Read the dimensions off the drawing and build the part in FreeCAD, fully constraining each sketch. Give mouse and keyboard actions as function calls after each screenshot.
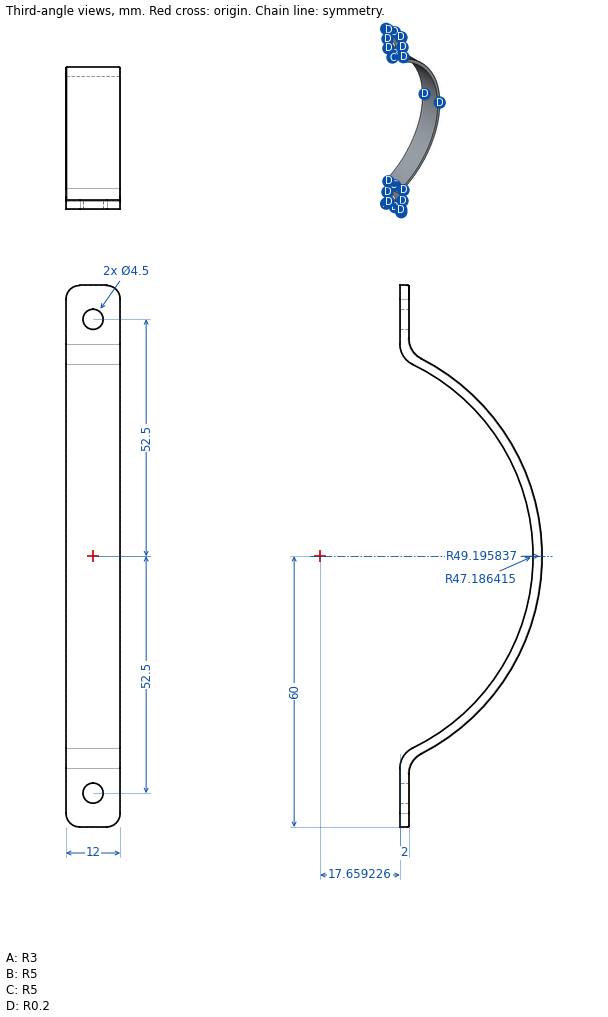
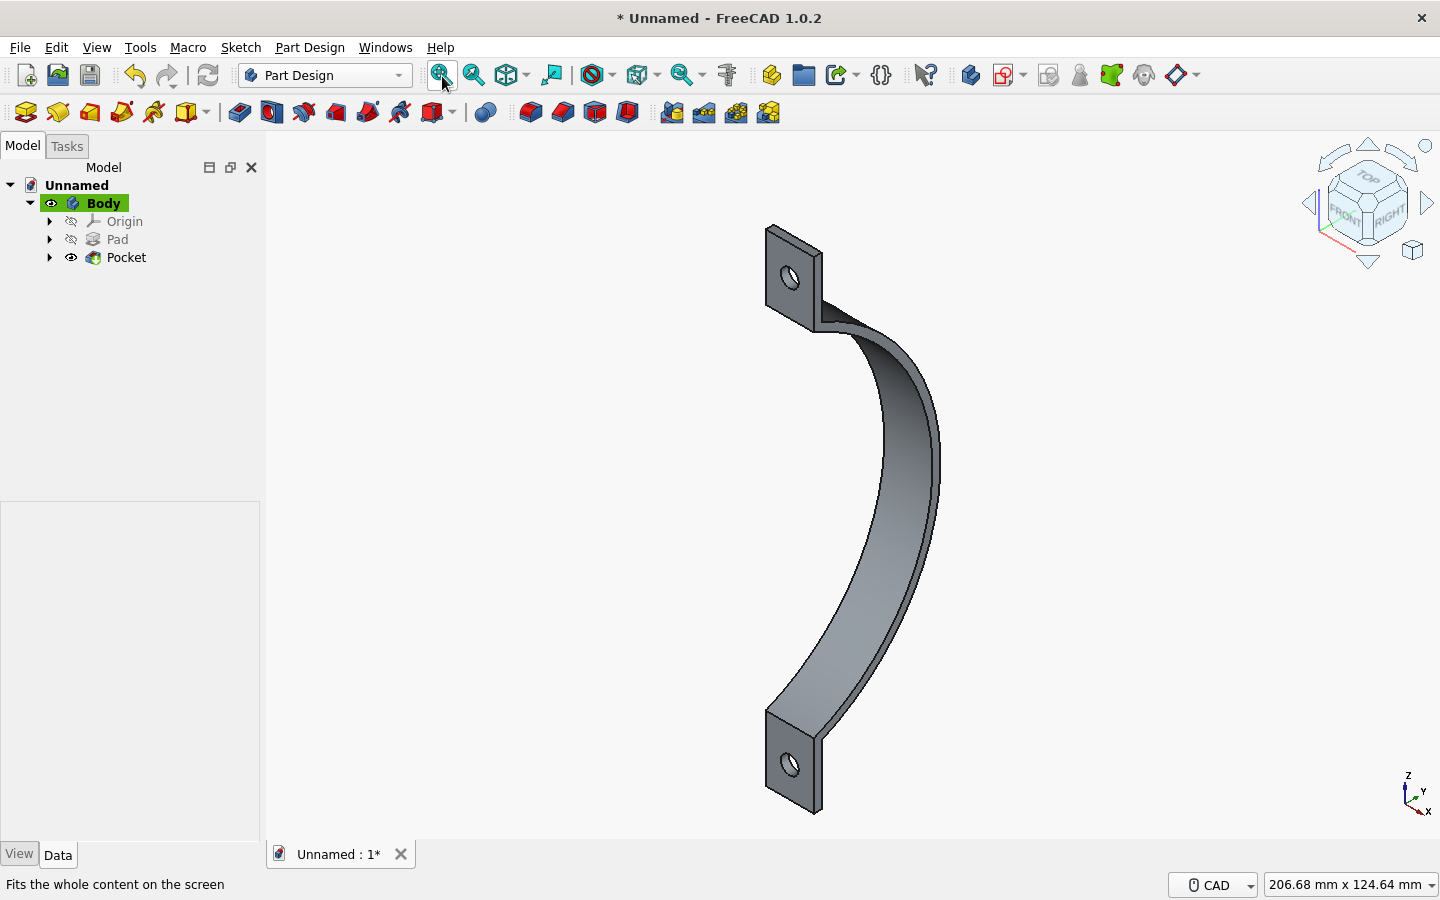
key(2)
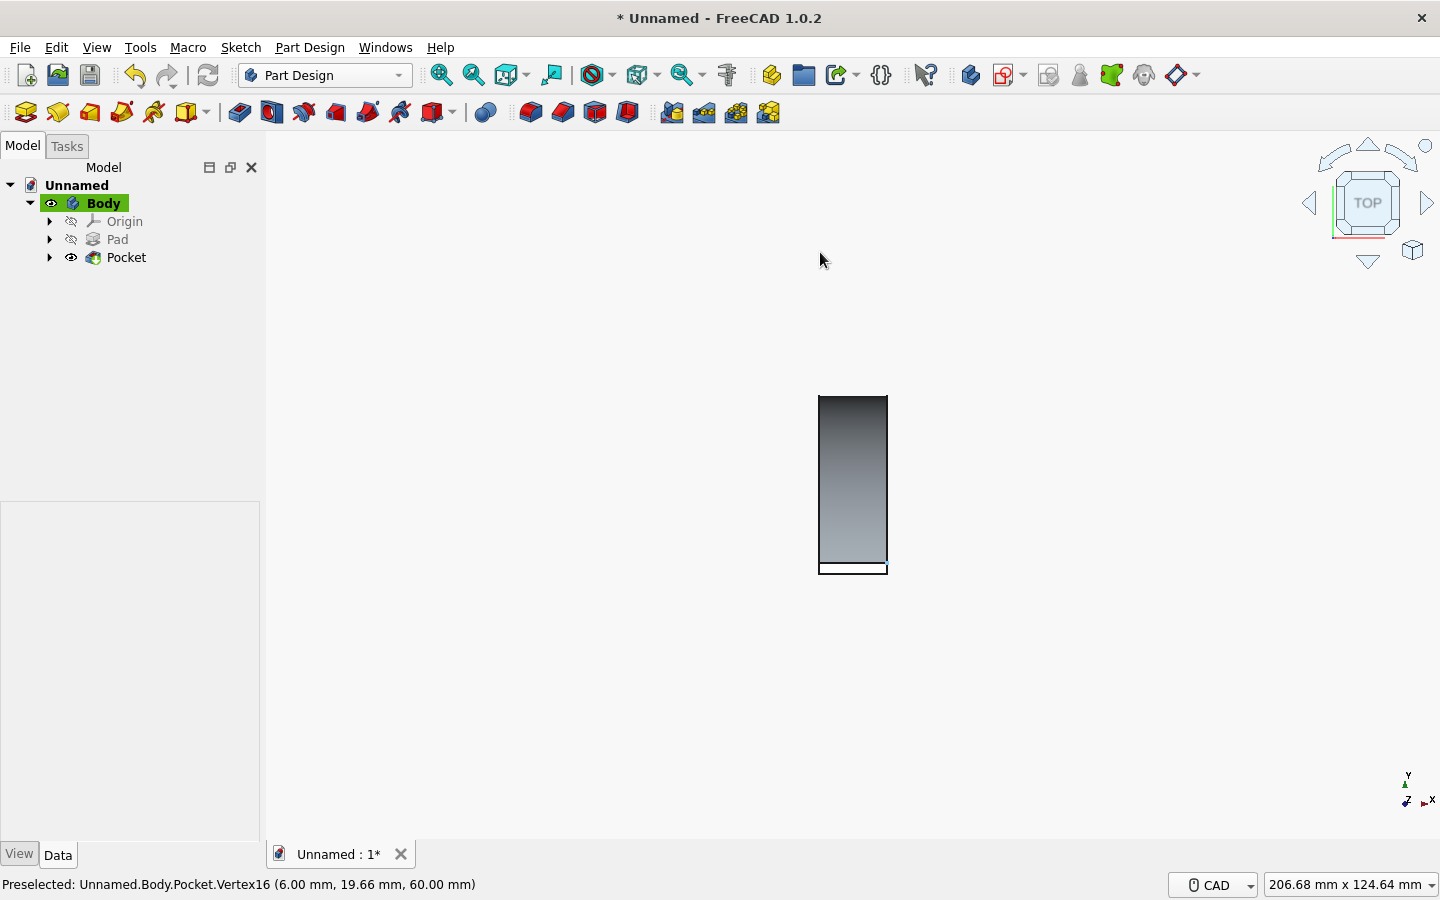
key(v)
key(f)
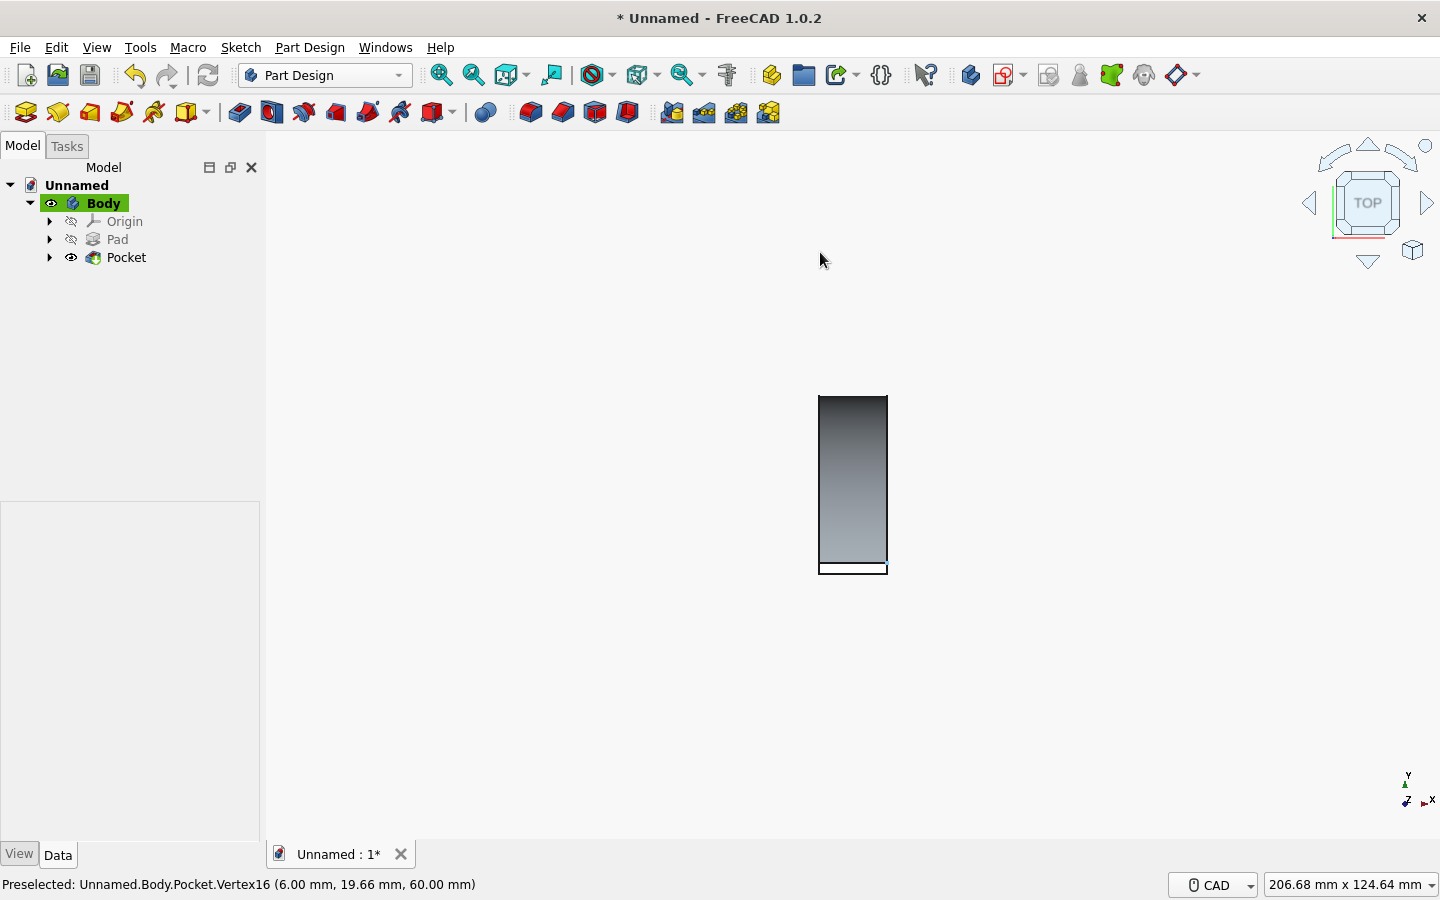
scroll(887, 568, up, 7)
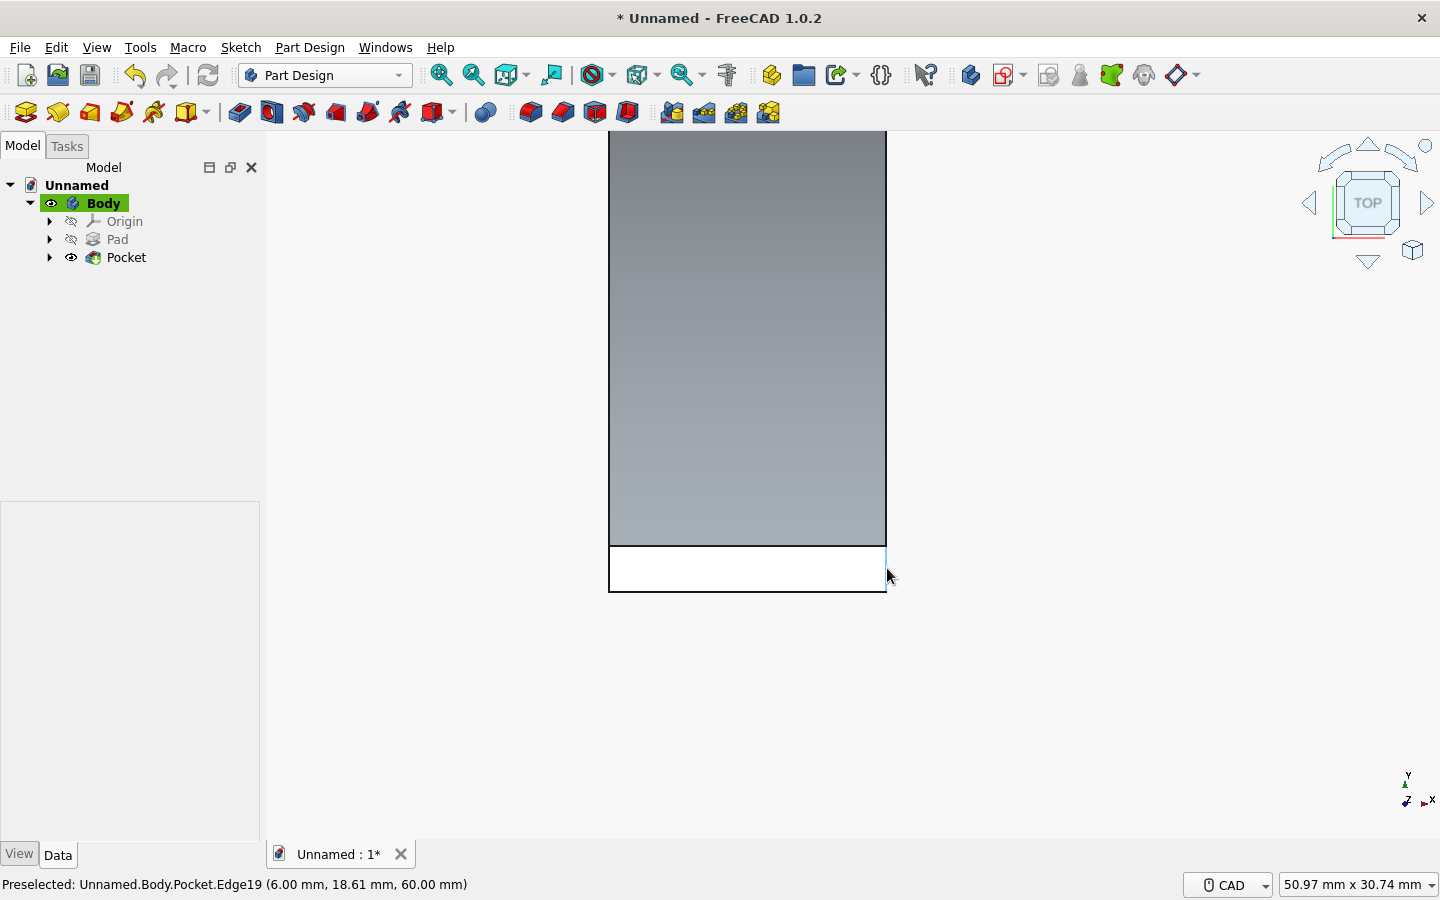
click(886, 568)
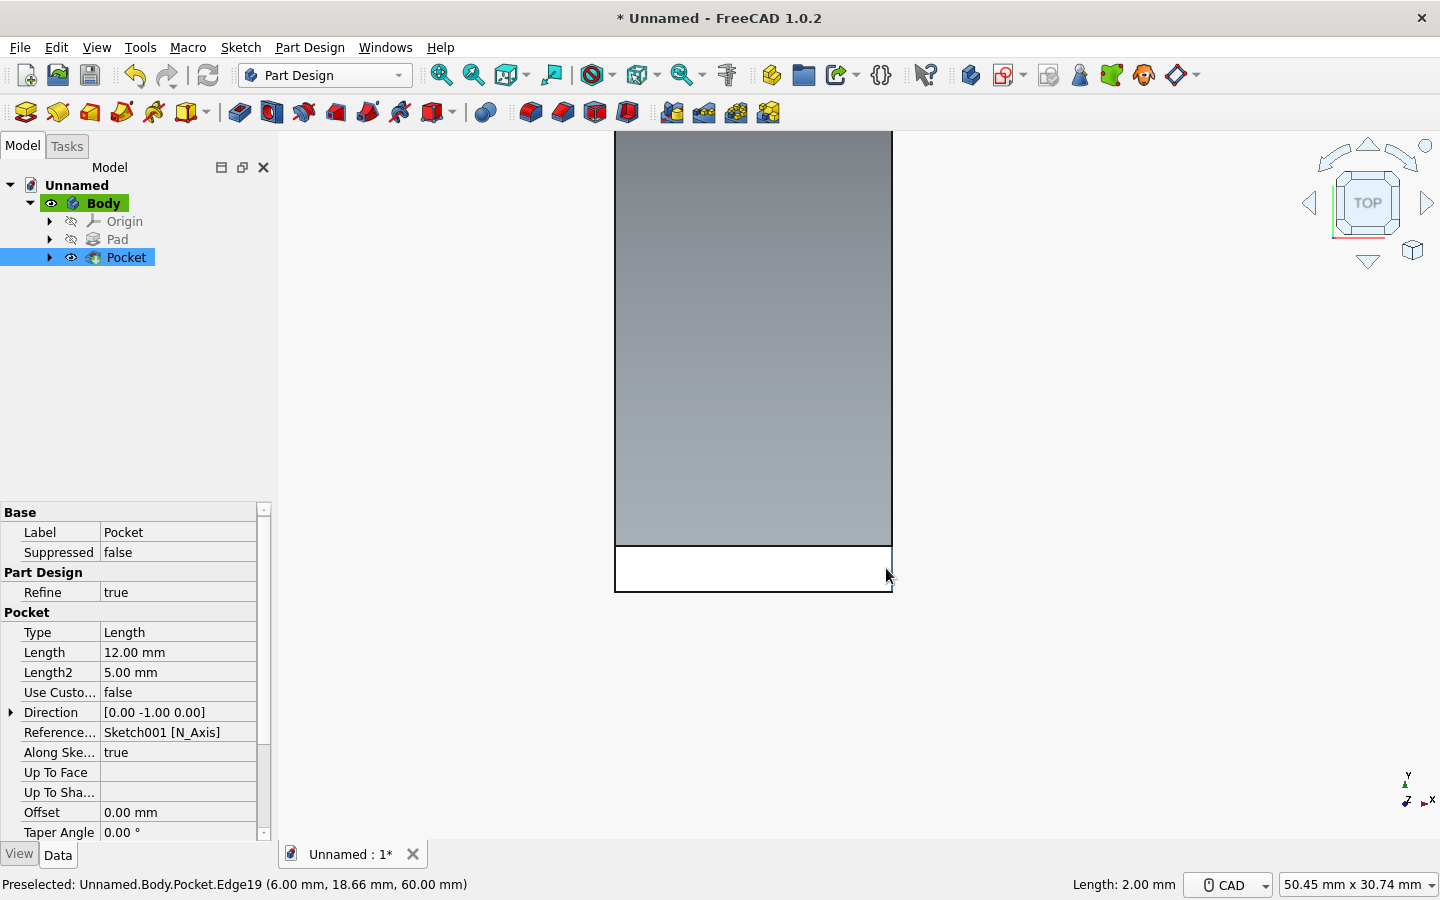
click(615, 568, ctrl)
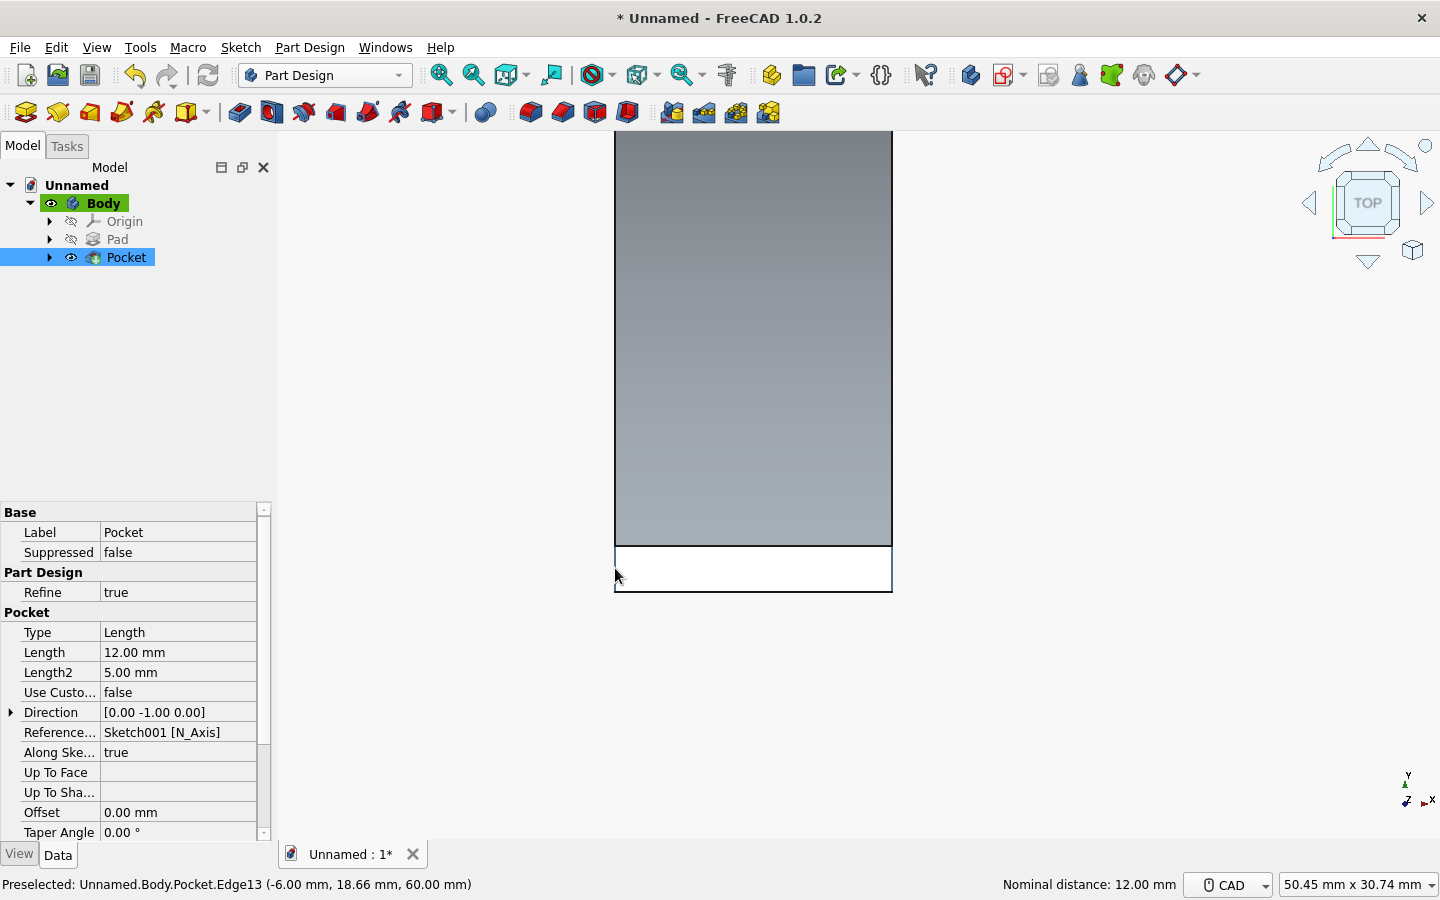
click(442, 76)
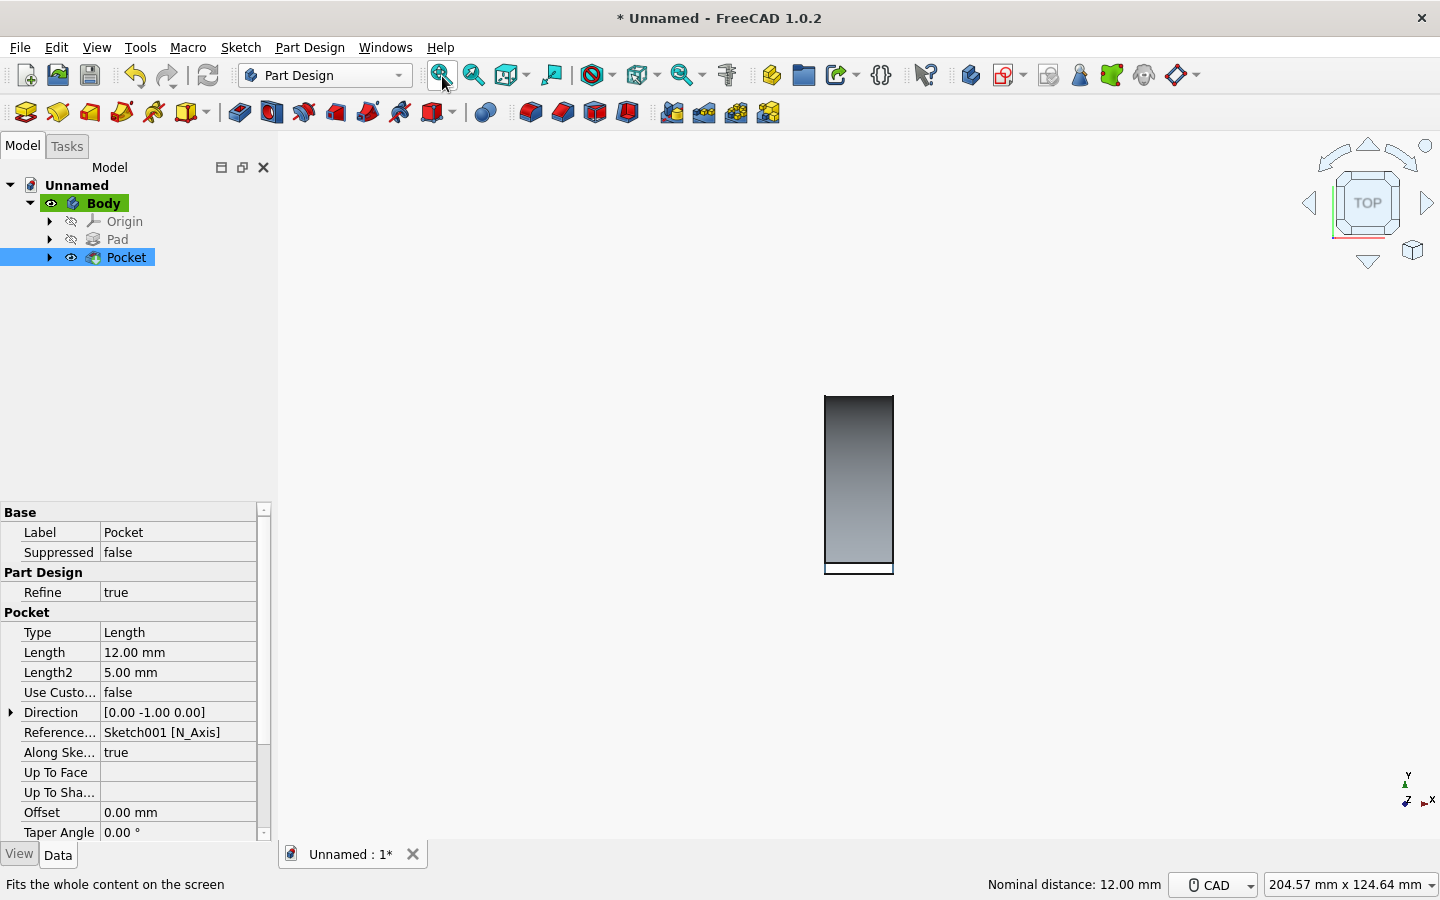
key(1)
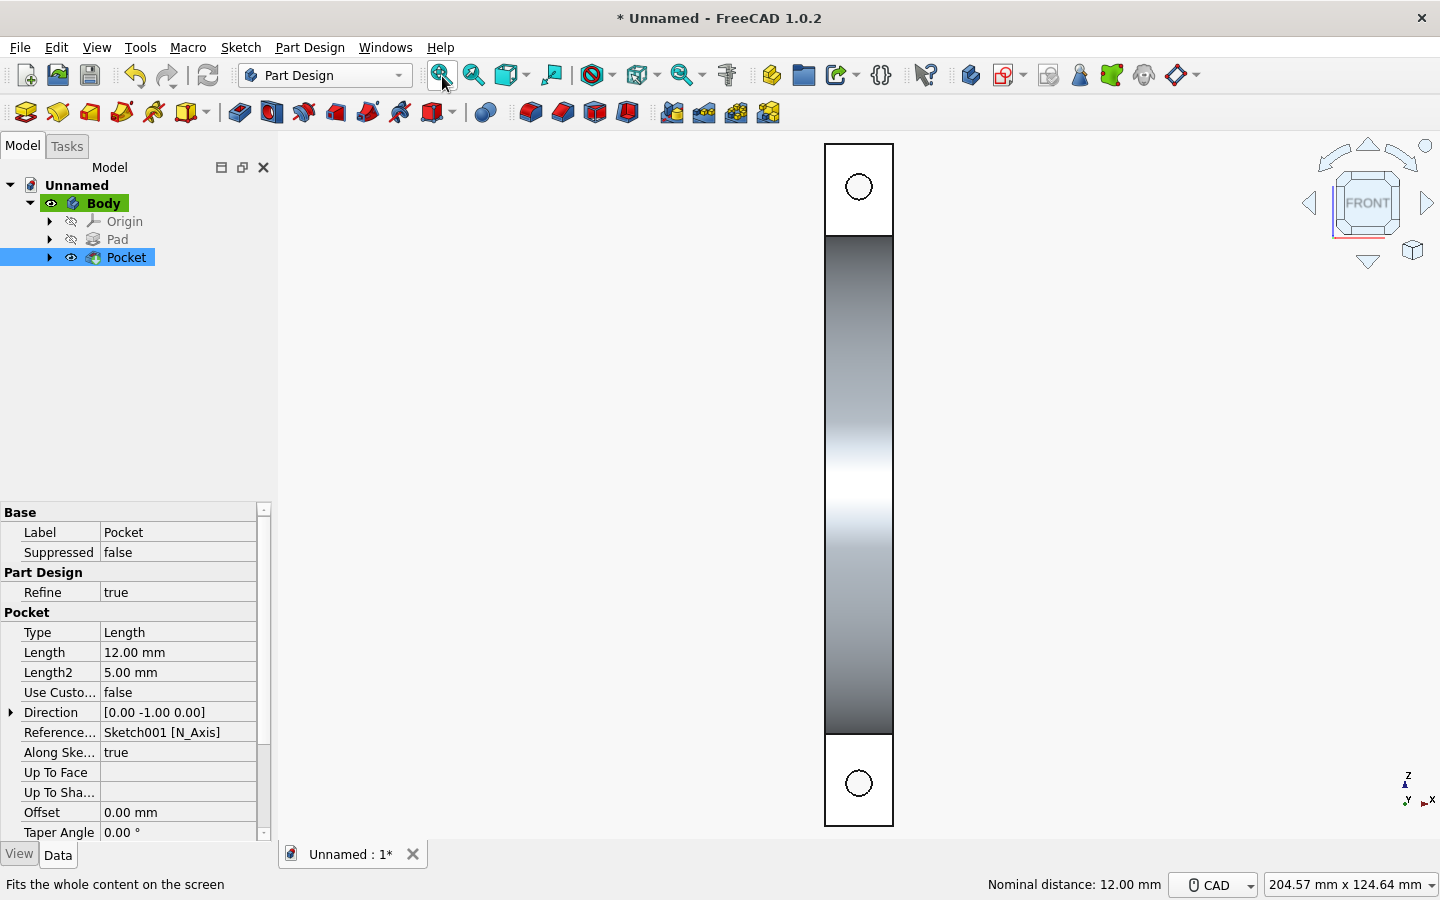
key(3)